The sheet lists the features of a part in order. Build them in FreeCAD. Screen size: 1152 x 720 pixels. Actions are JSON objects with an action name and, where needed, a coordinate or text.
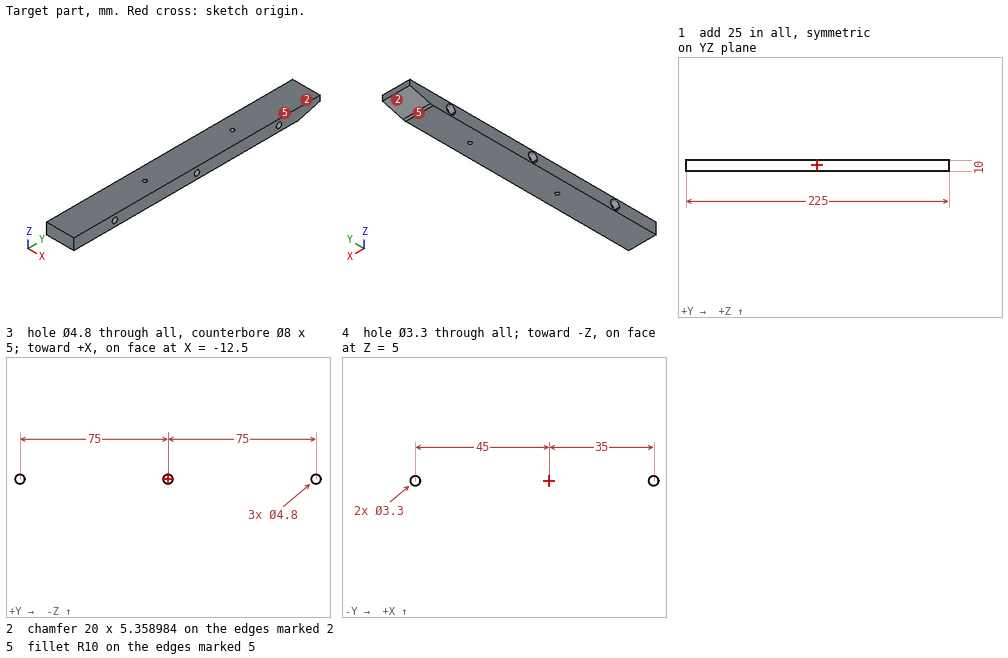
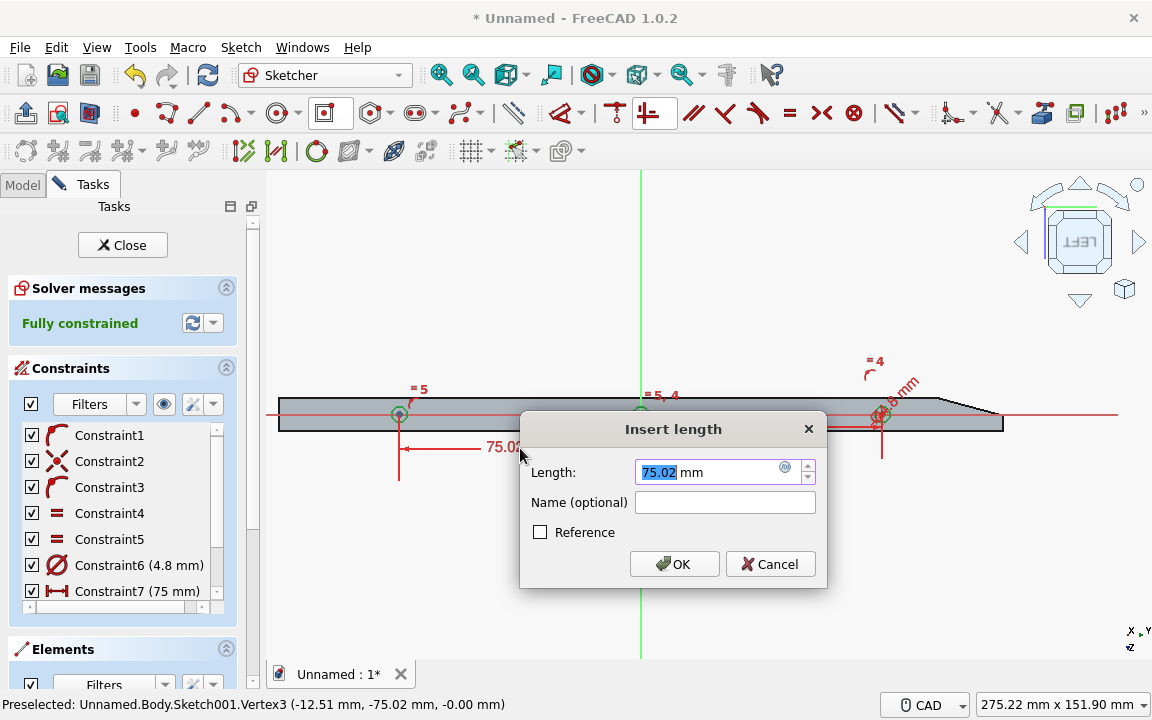
{"action": "type", "text": "75"}
{"action": "key", "text": "Return"}
{"action": "key", "text": "Escape"}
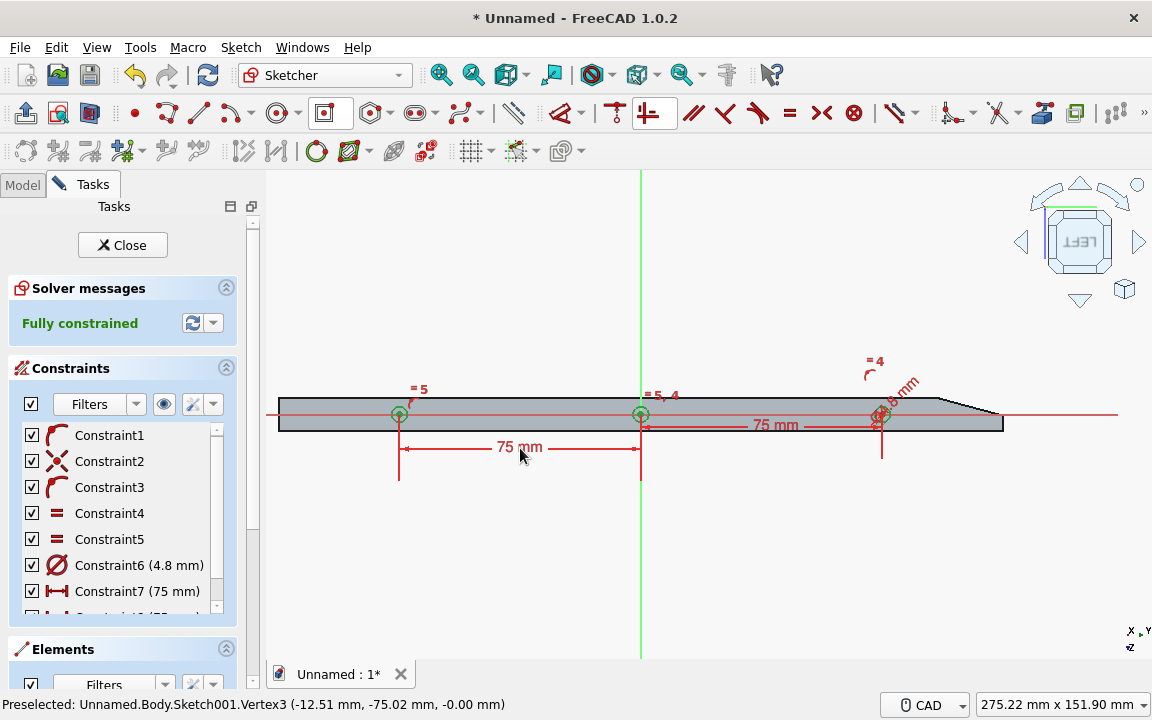
{"action": "left_click", "coordinate": [123, 245]}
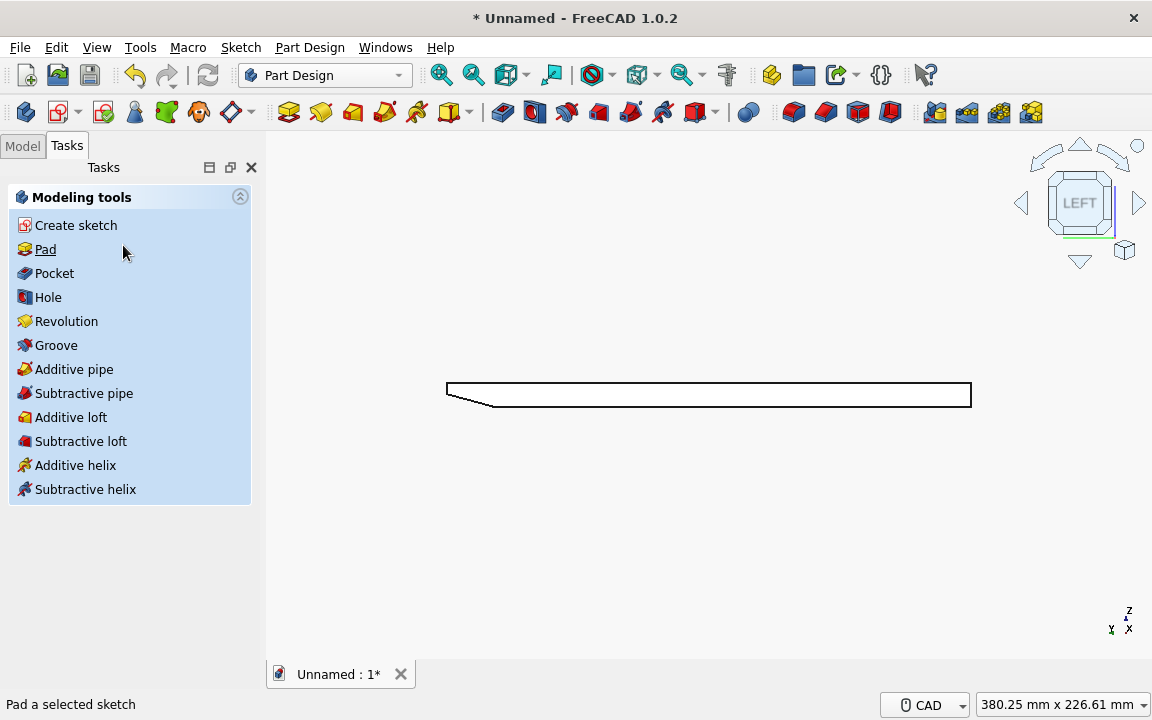
{"action": "left_click", "coordinate": [536, 112]}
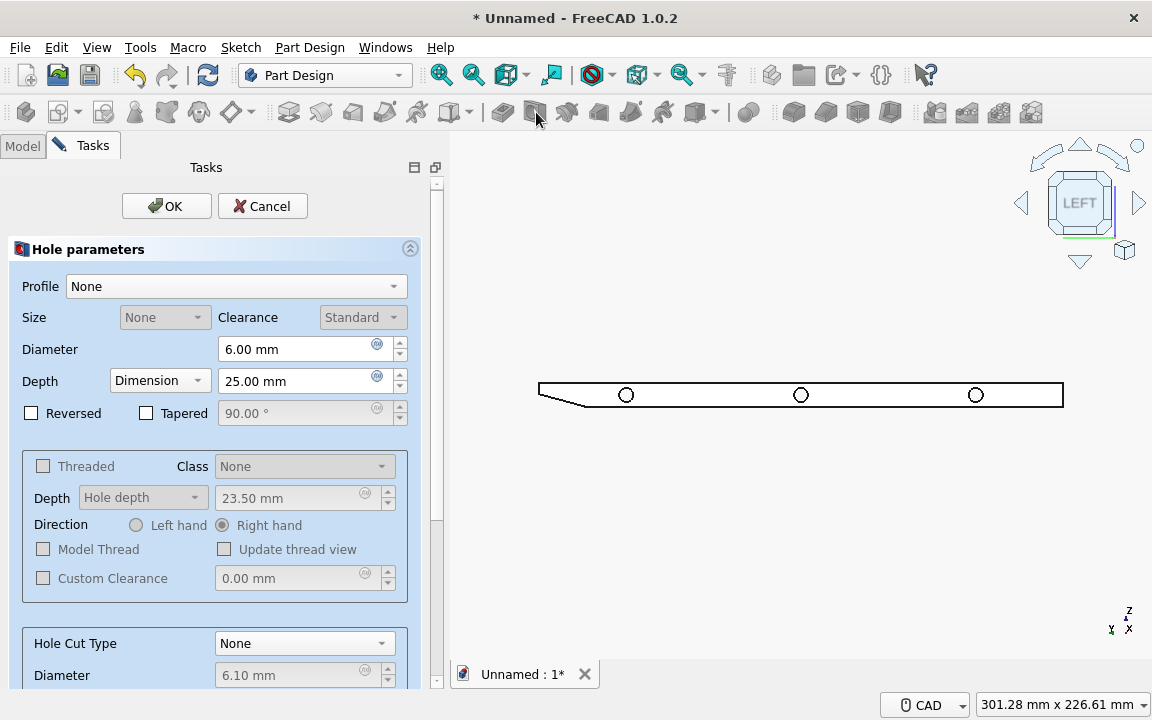
{"action": "triple_click", "coordinate": [305, 349]}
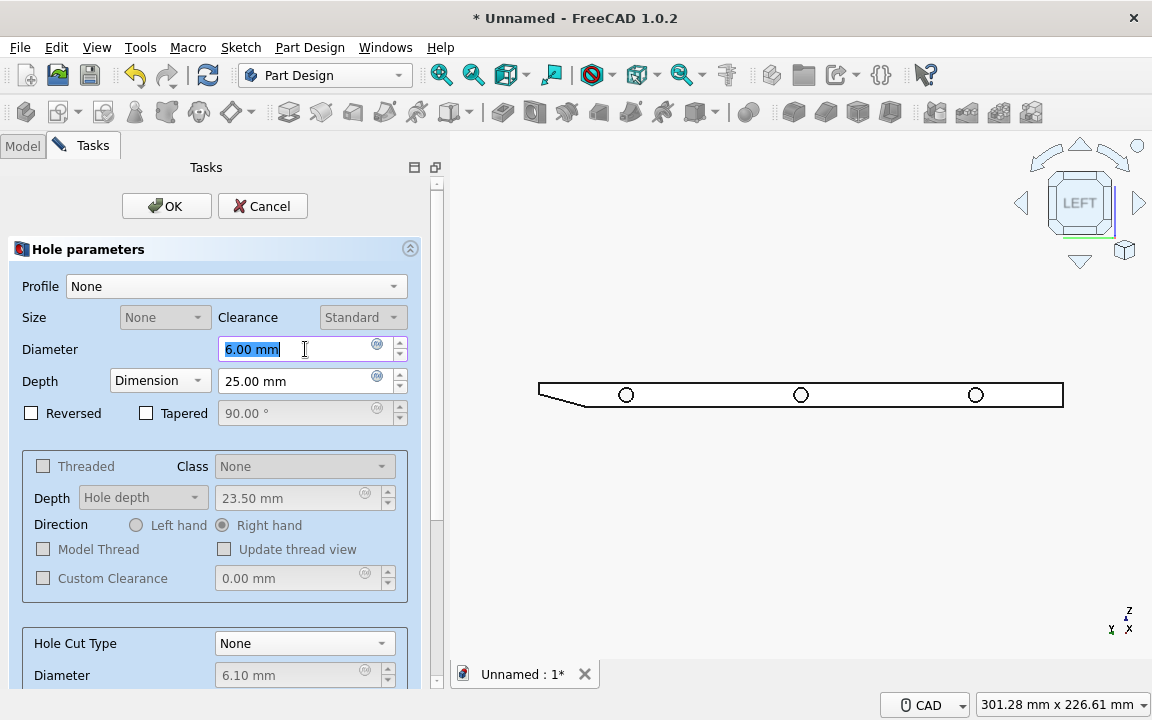
{"action": "type", "text": "4.8"}
{"action": "key", "text": "Tab"}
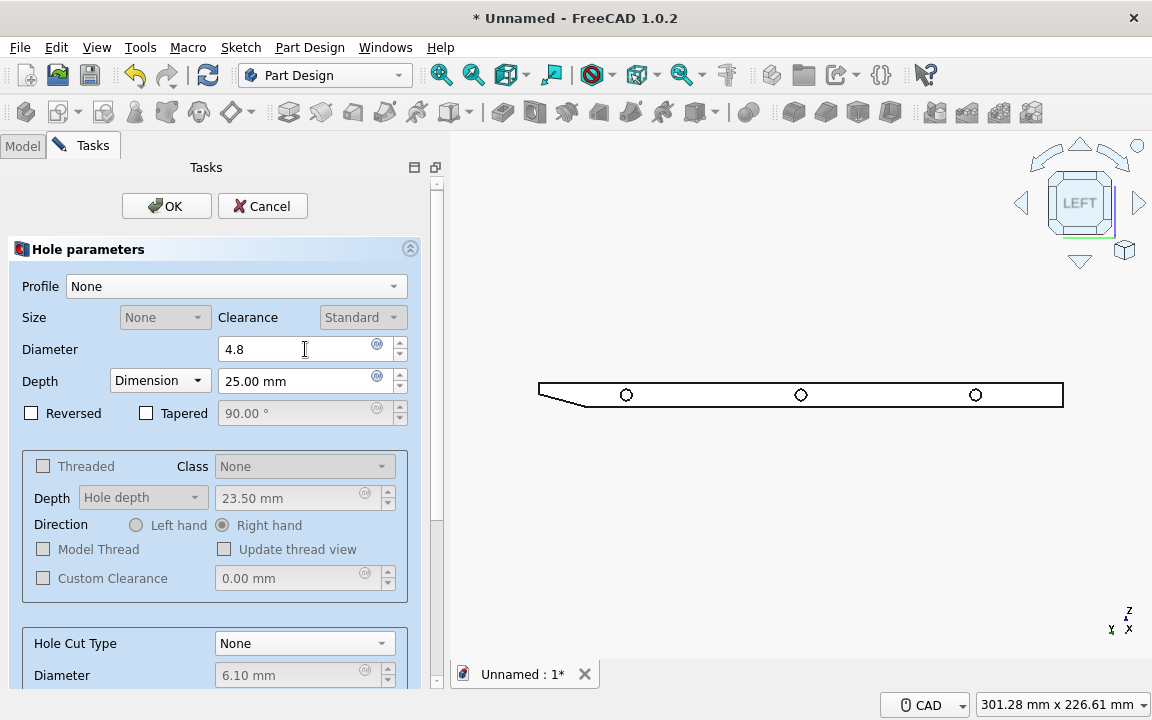
{"action": "left_click", "coordinate": [161, 380]}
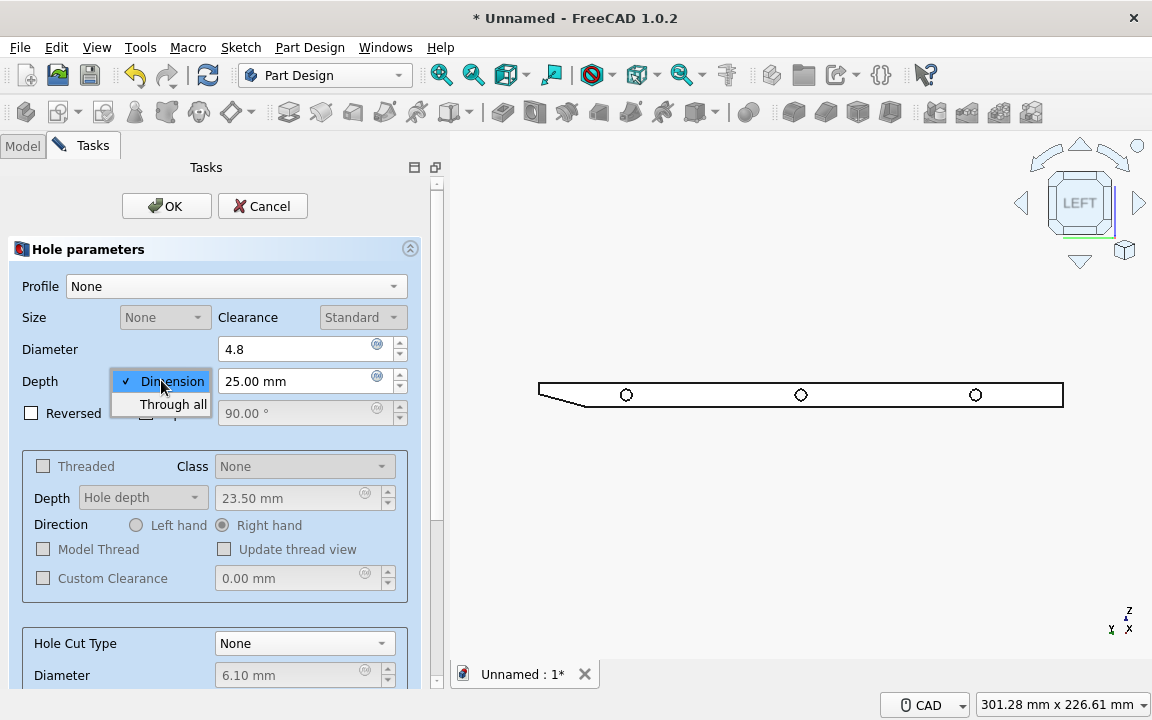
{"action": "left_click", "coordinate": [160, 404]}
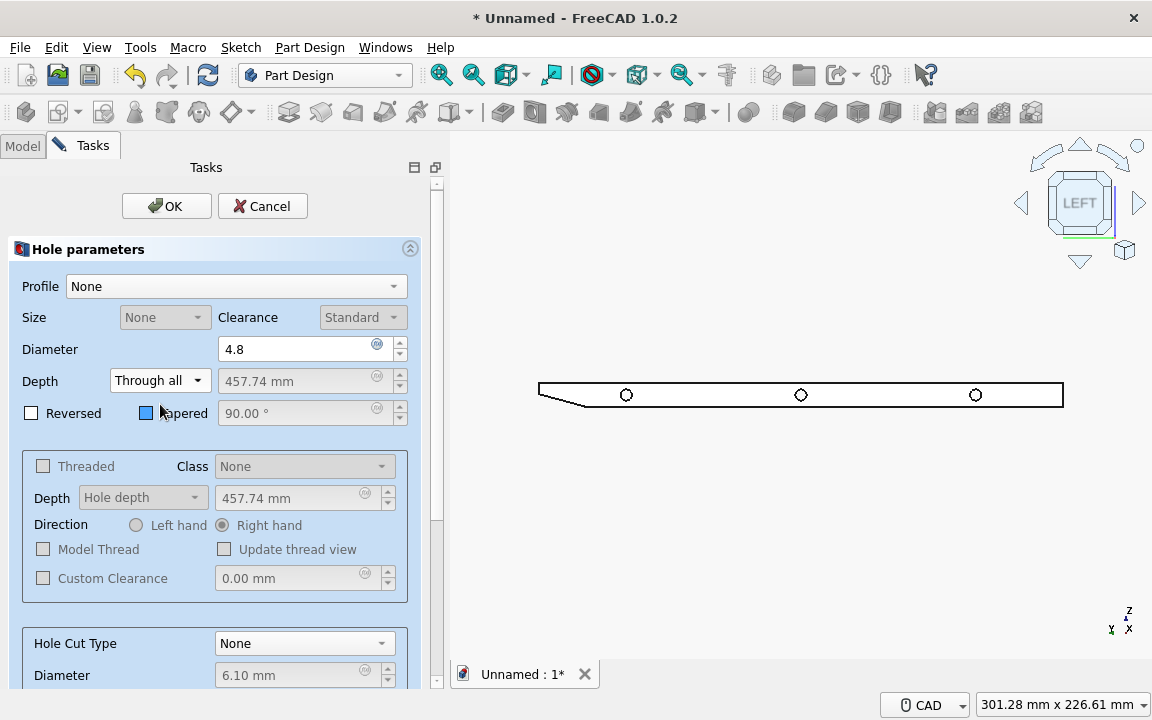
{"action": "left_click", "coordinate": [306, 644]}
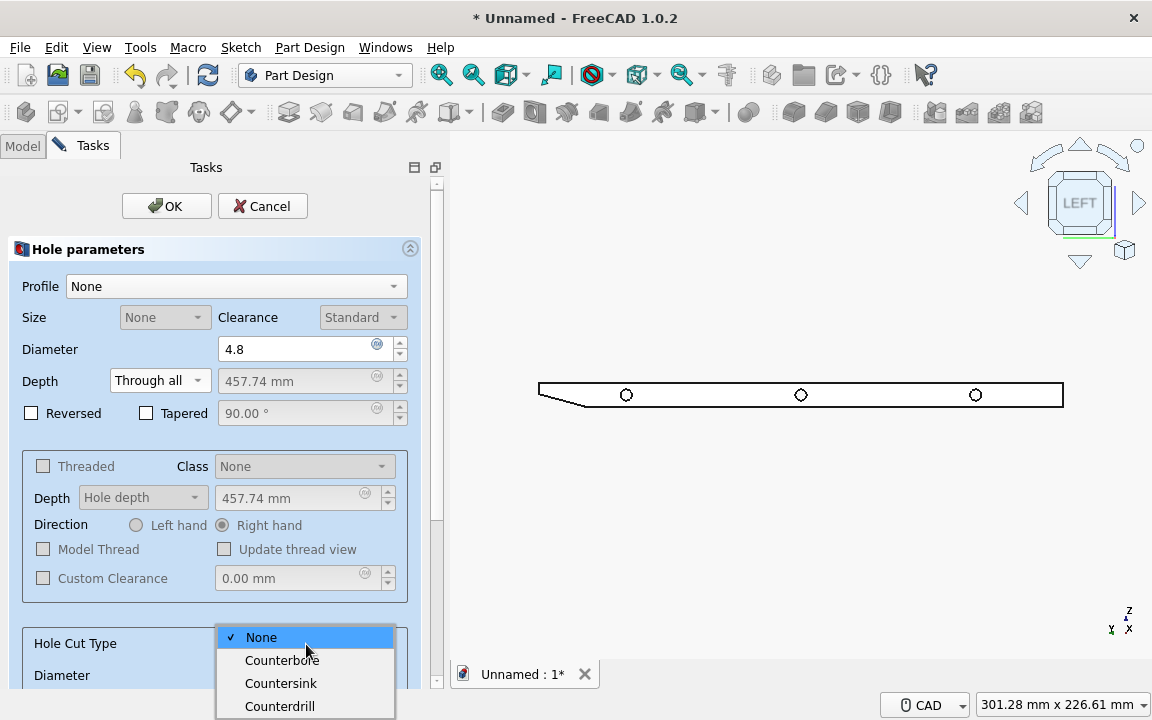
{"action": "left_click", "coordinate": [304, 660]}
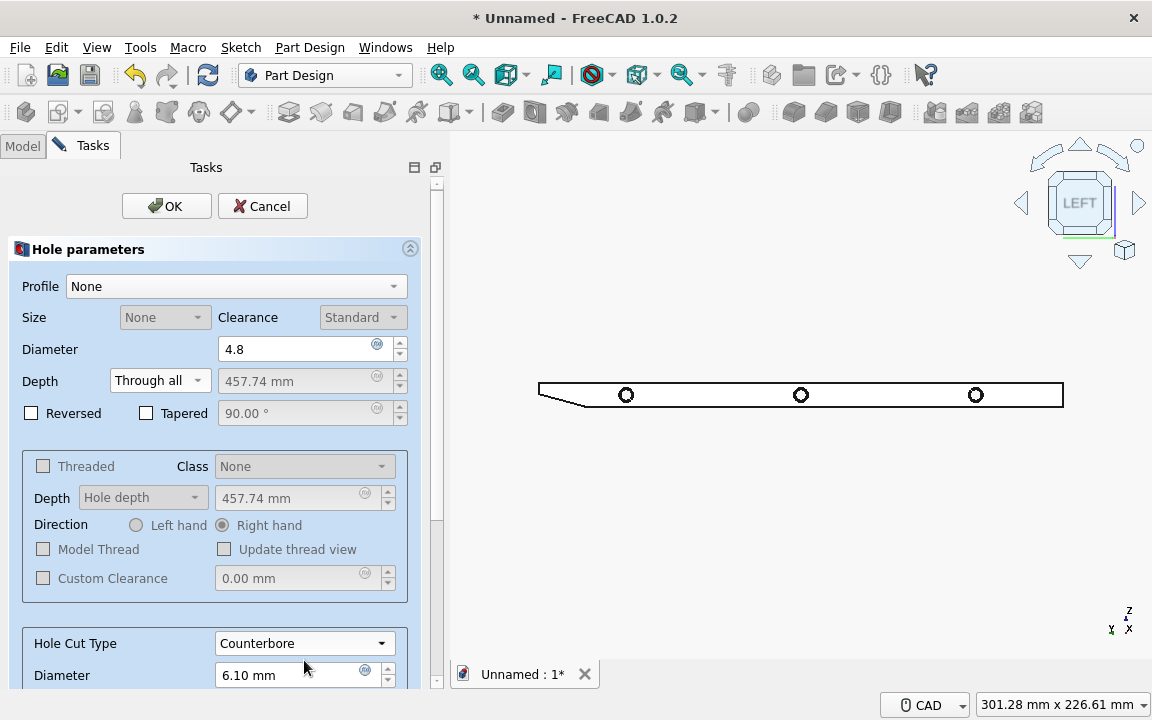
{"action": "triple_click", "coordinate": [298, 675]}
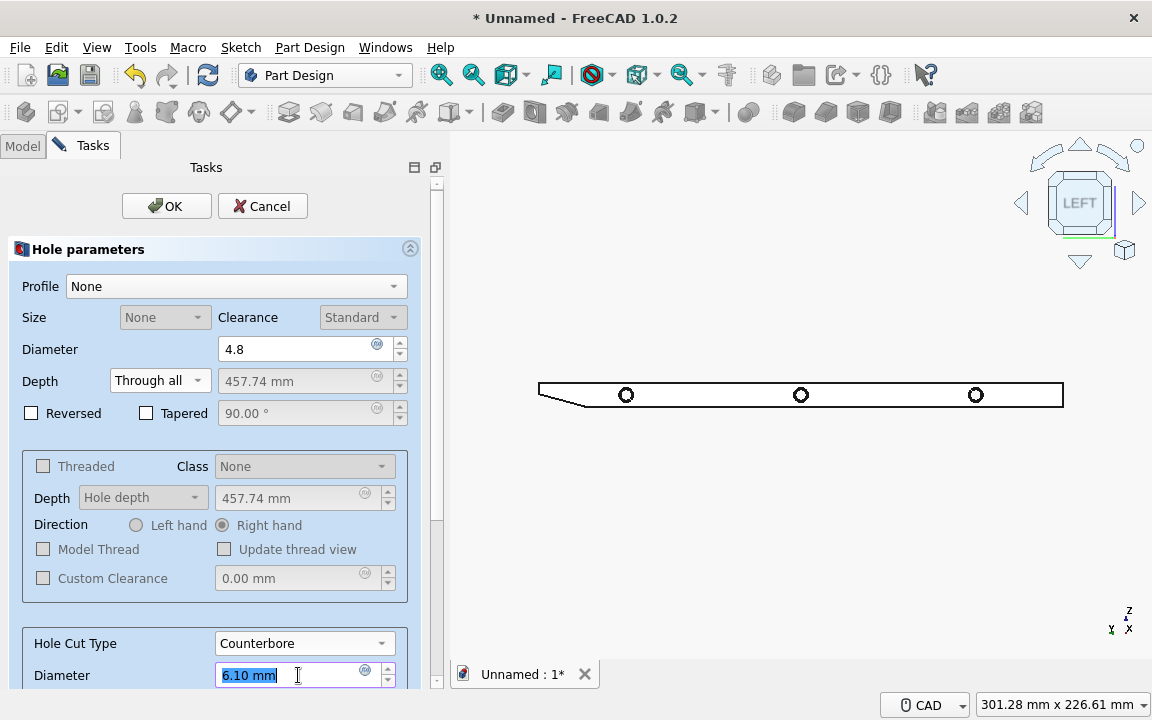
{"action": "type", "text": "8"}
{"action": "key", "text": "Tab"}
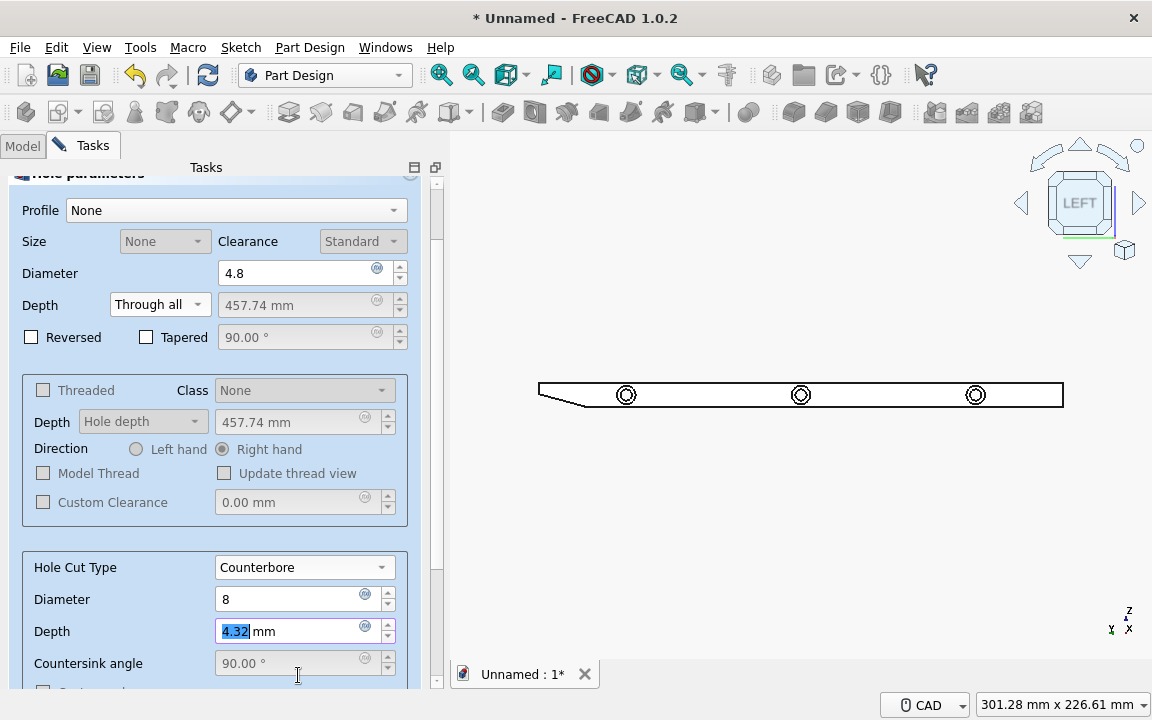
{"action": "type", "text": "5"}
{"action": "key", "text": "Tab"}